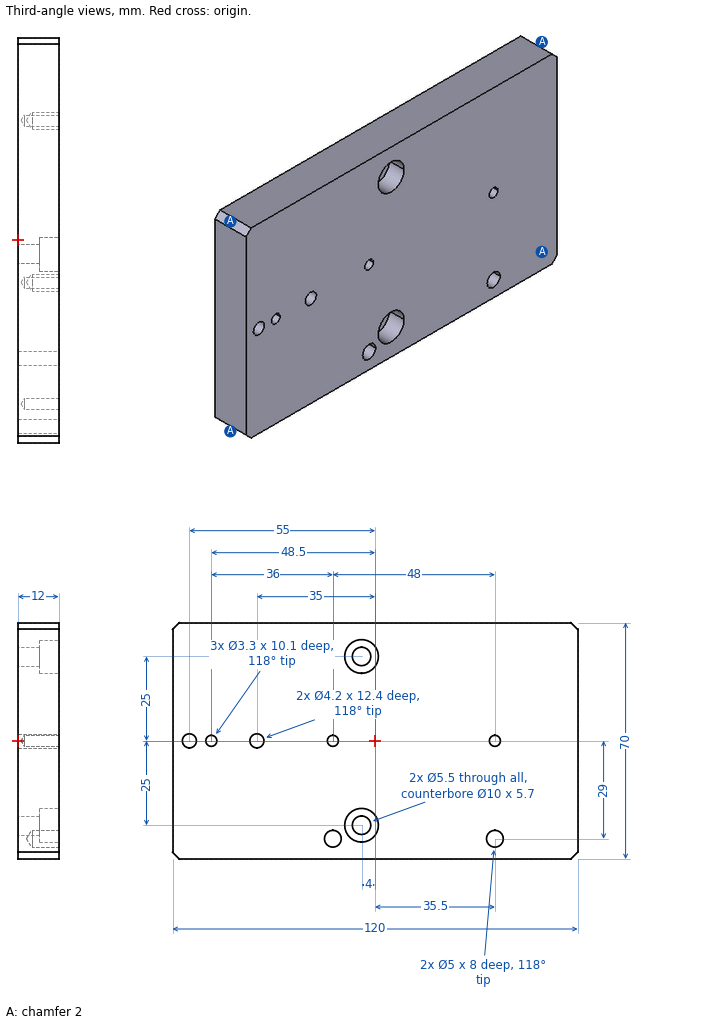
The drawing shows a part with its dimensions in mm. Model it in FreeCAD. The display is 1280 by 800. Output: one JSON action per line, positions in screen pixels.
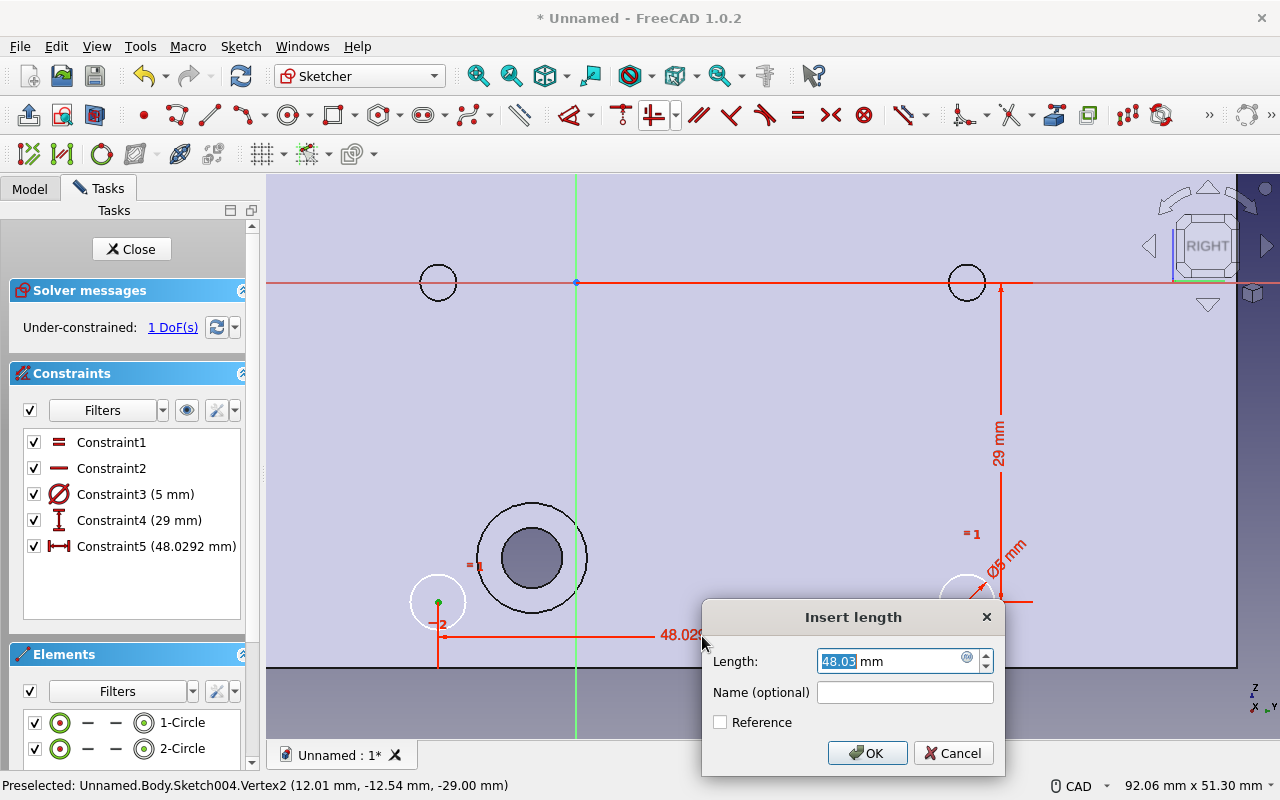
{"action": "type", "text": "48"}
{"action": "key", "text": "Return"}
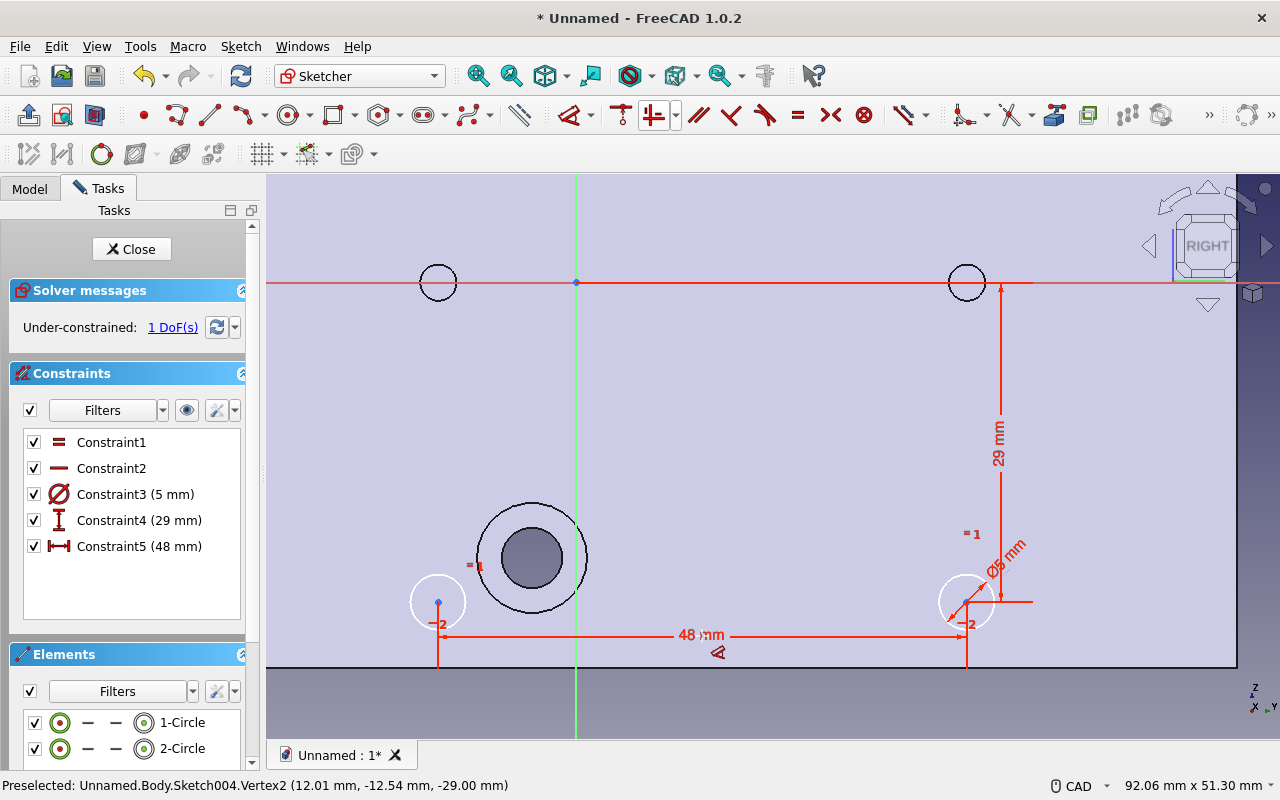
{"action": "left_click", "coordinate": [967, 602]}
{"action": "left_click", "coordinate": [771, 249]}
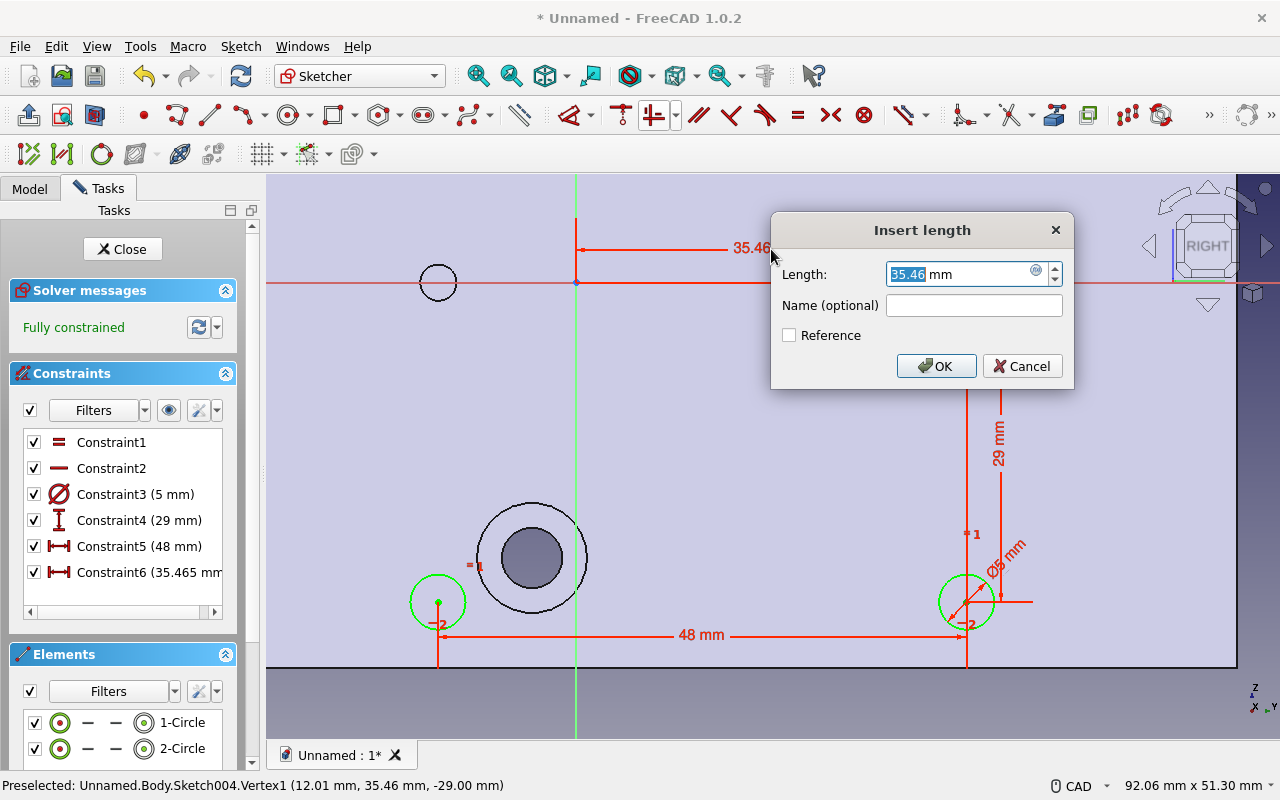
{"action": "type", "text": "35.5"}
{"action": "key", "text": "Return"}
{"action": "key", "text": "Escape"}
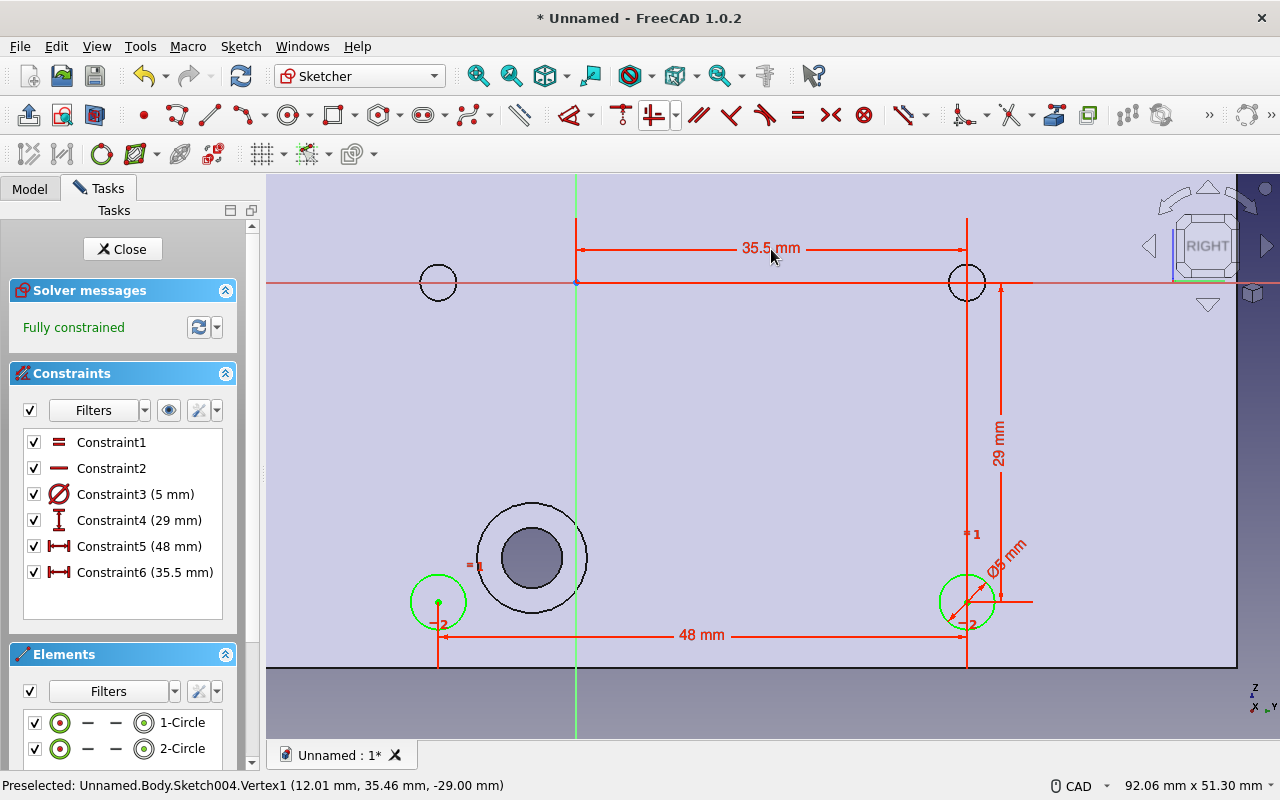
{"action": "left_click", "coordinate": [123, 249]}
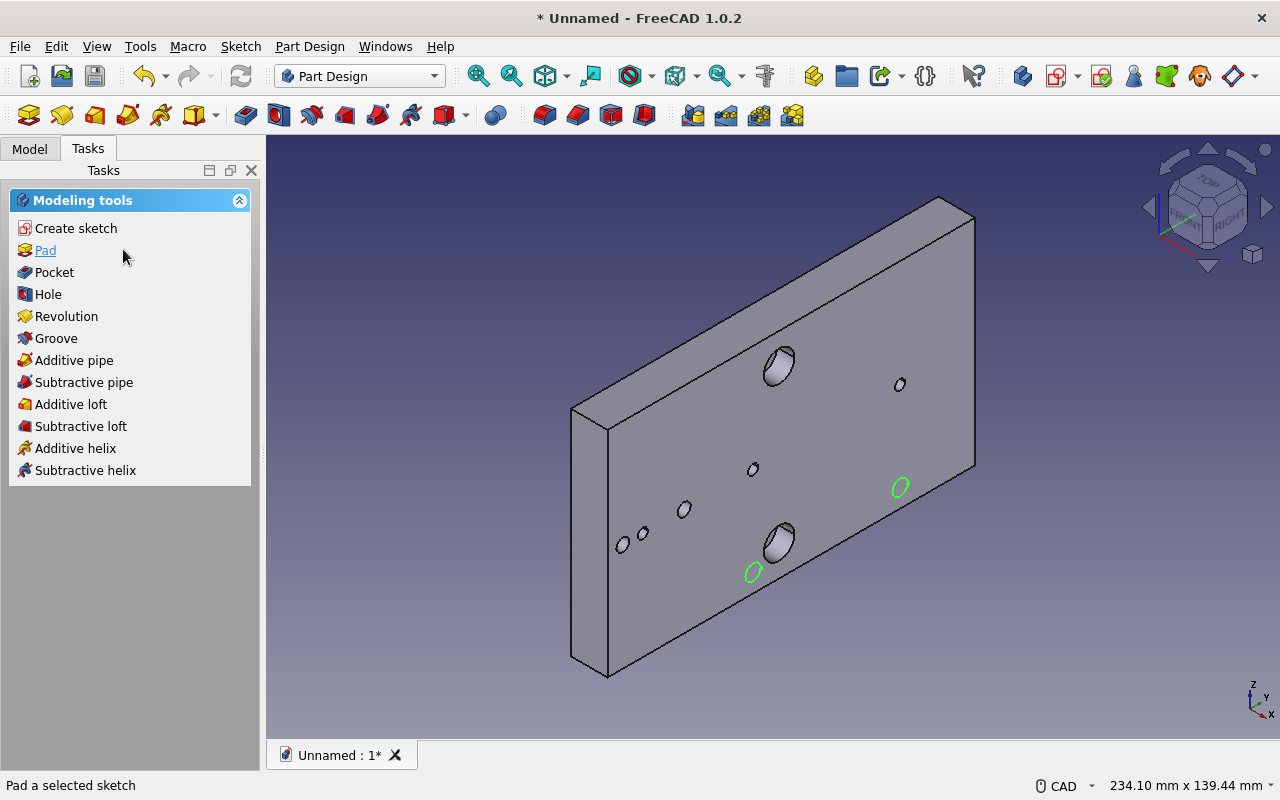
{"action": "left_click", "coordinate": [279, 116]}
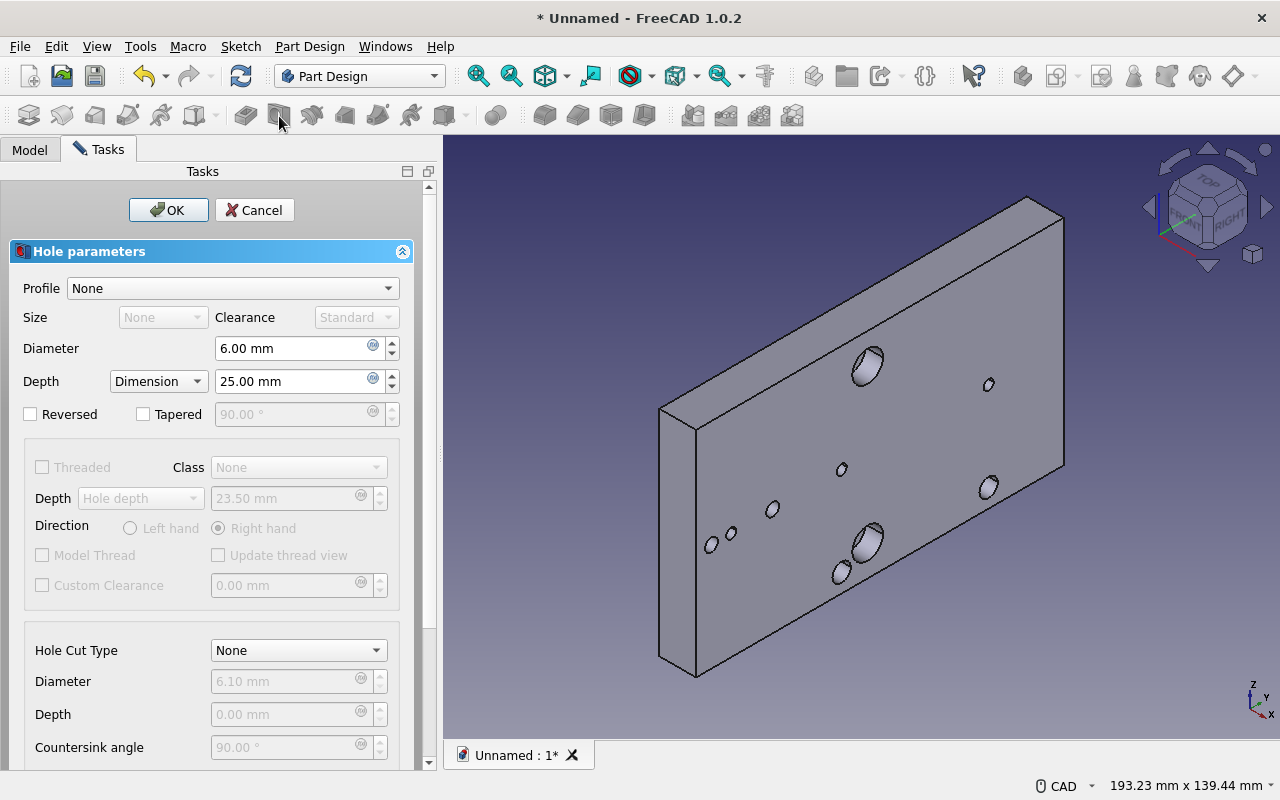
{"action": "triple_click", "coordinate": [300, 348]}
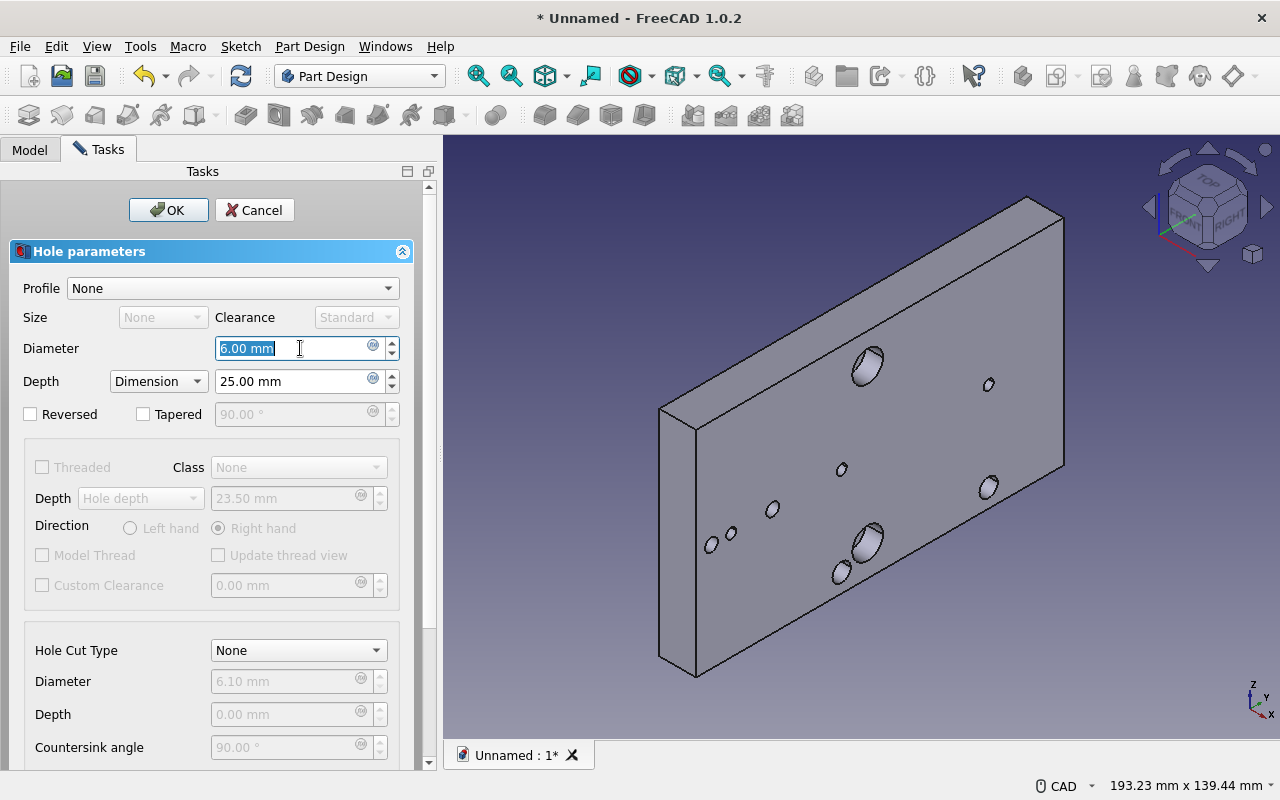
{"action": "type", "text": "5"}
{"action": "key", "text": "Tab"}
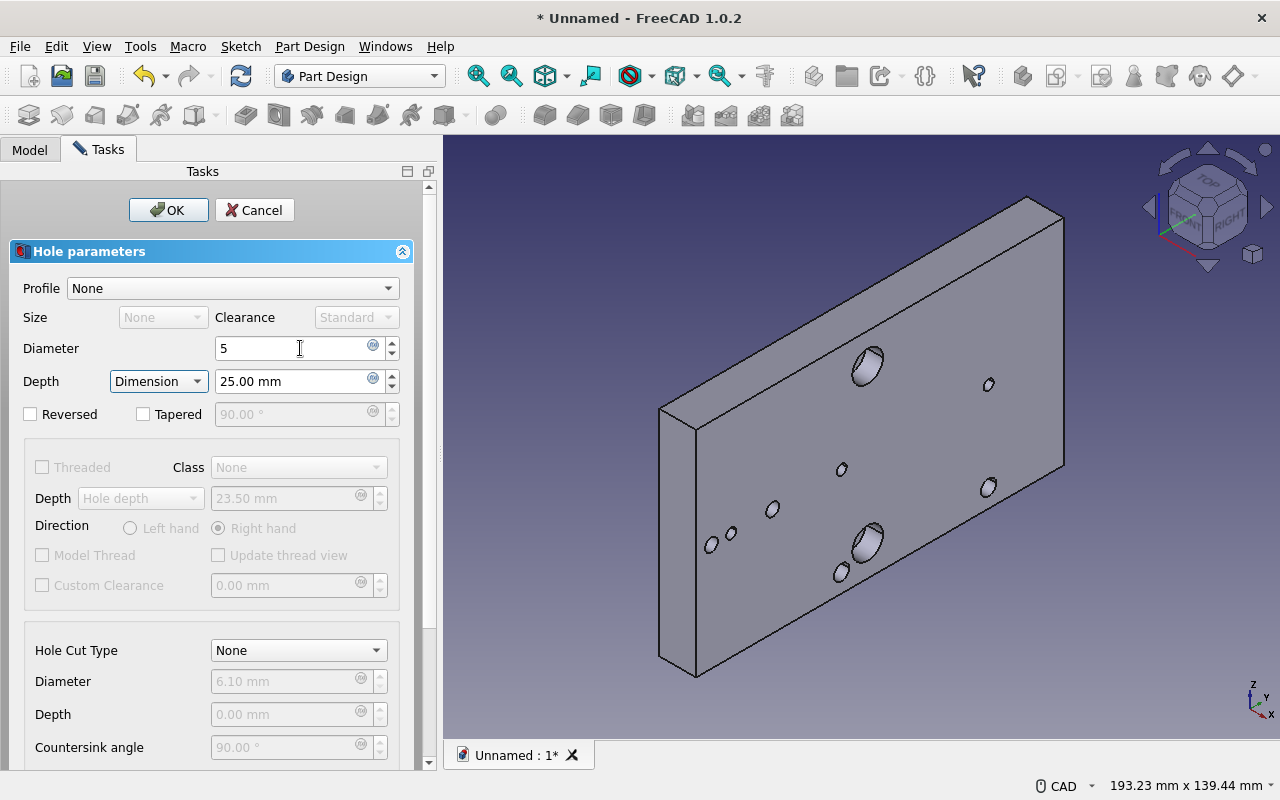
{"action": "triple_click", "coordinate": [300, 382]}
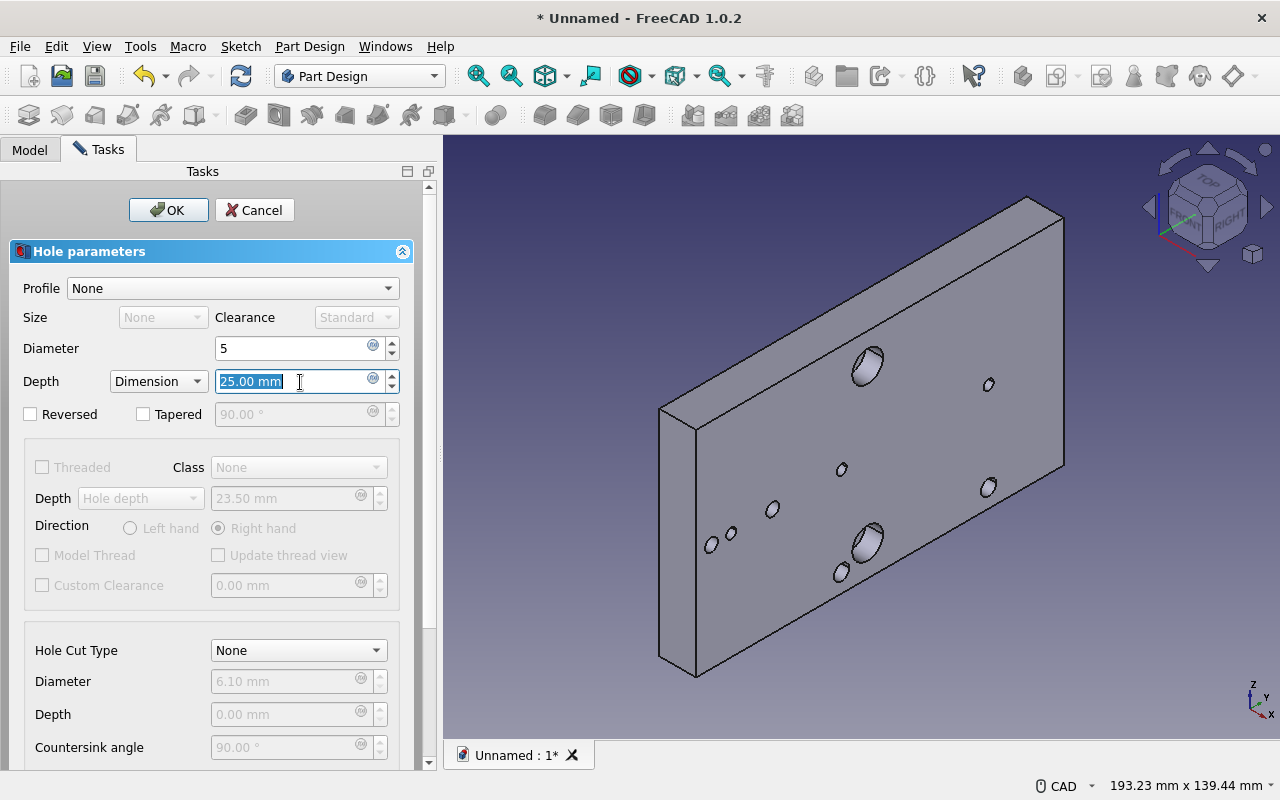
{"action": "type", "text": "8"}
{"action": "key", "text": "Tab"}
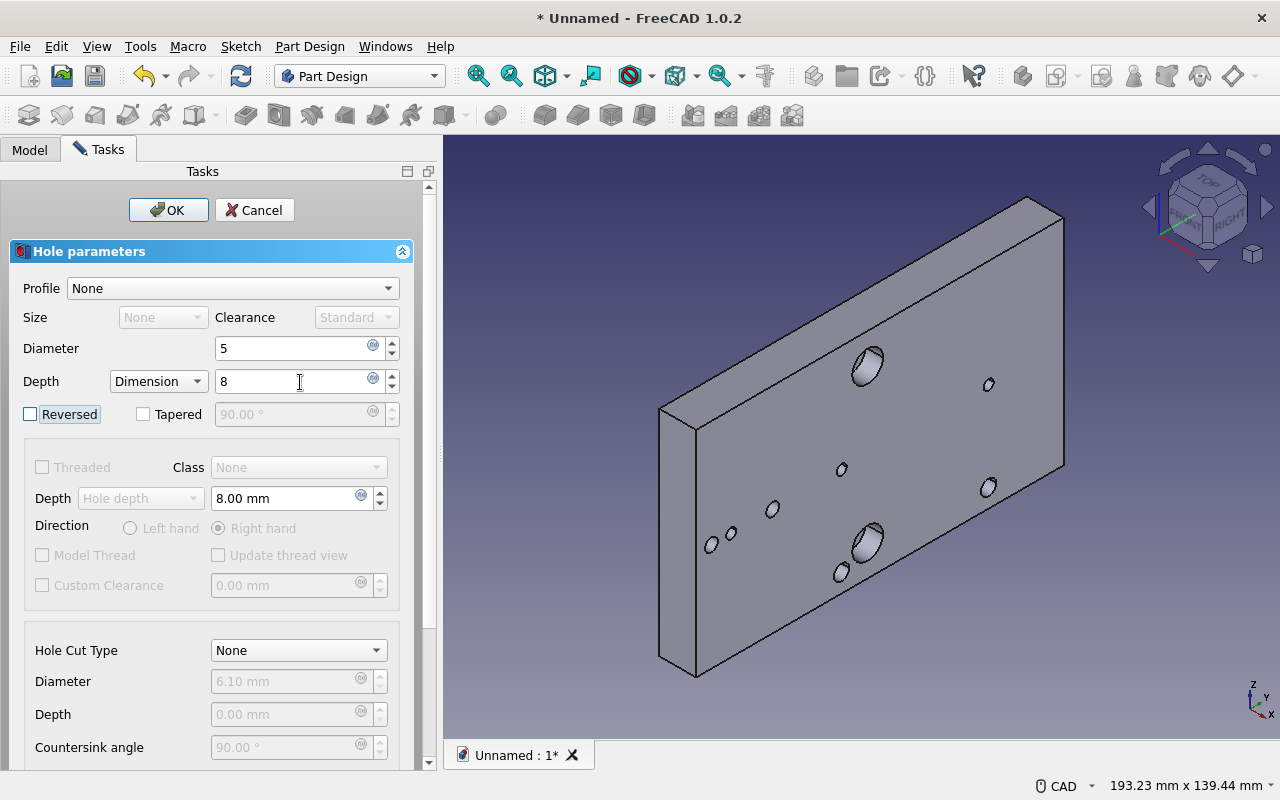
{"action": "left_click", "coordinate": [169, 210]}